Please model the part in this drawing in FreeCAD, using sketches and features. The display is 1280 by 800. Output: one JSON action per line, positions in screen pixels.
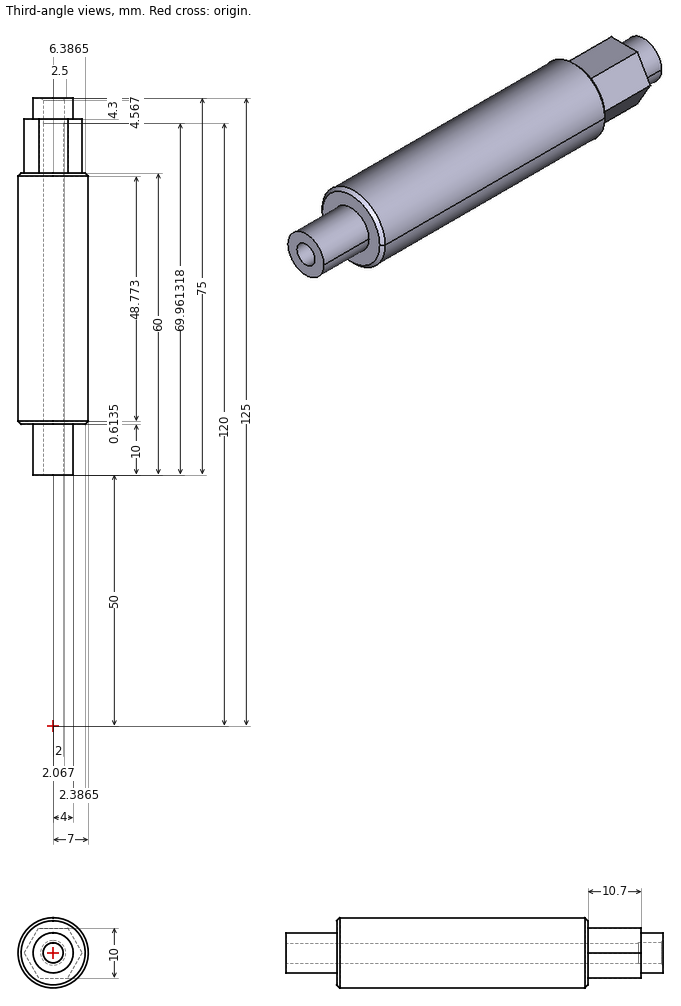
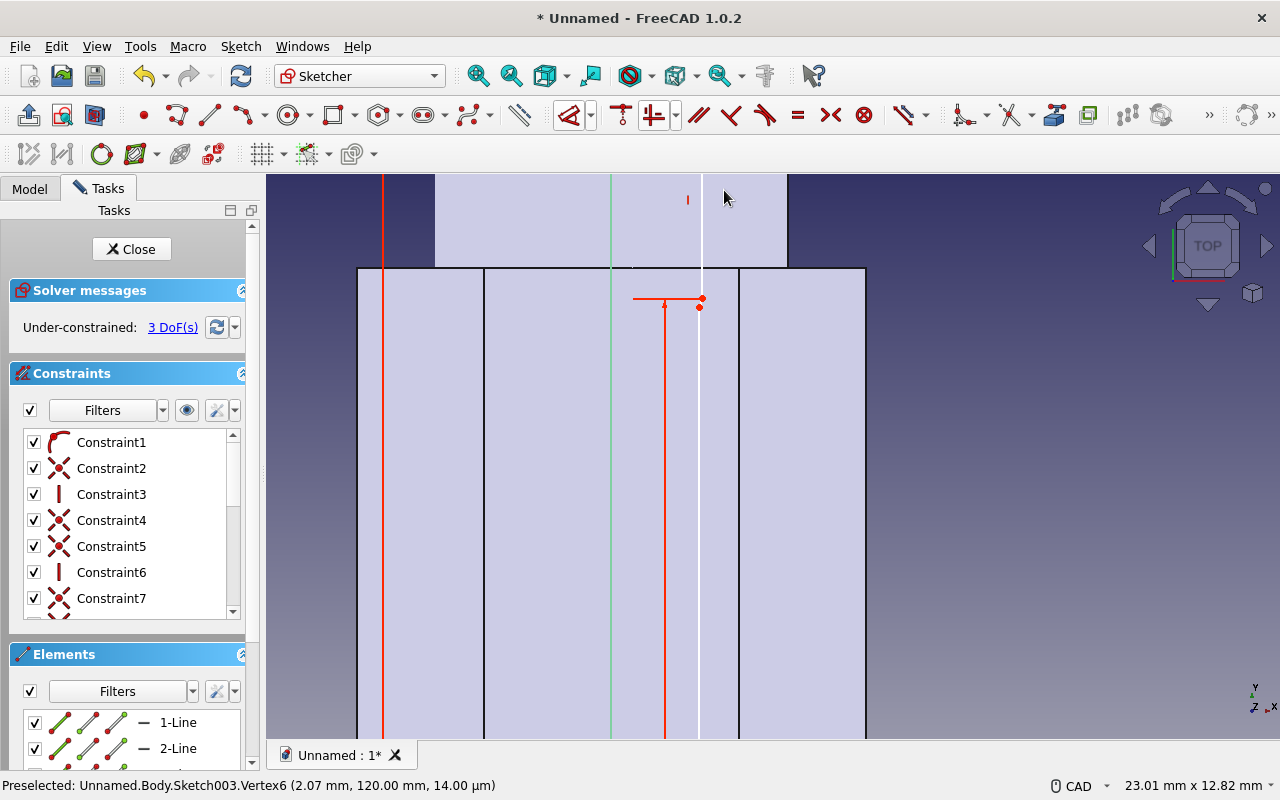
{"action": "scroll", "coordinate": [707, 303], "scroll_direction": "down", "scroll_amount": 14}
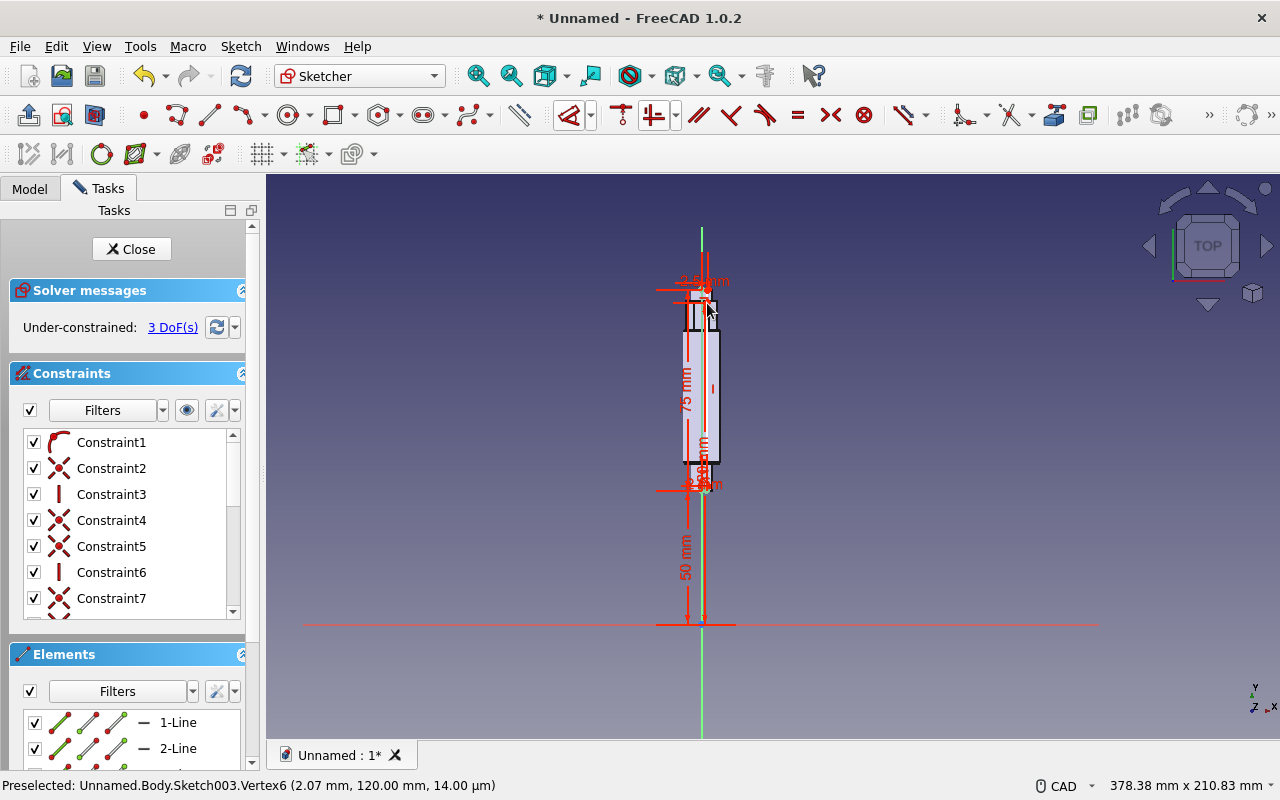
{"action": "scroll", "coordinate": [707, 299], "scroll_direction": "up", "scroll_amount": 7}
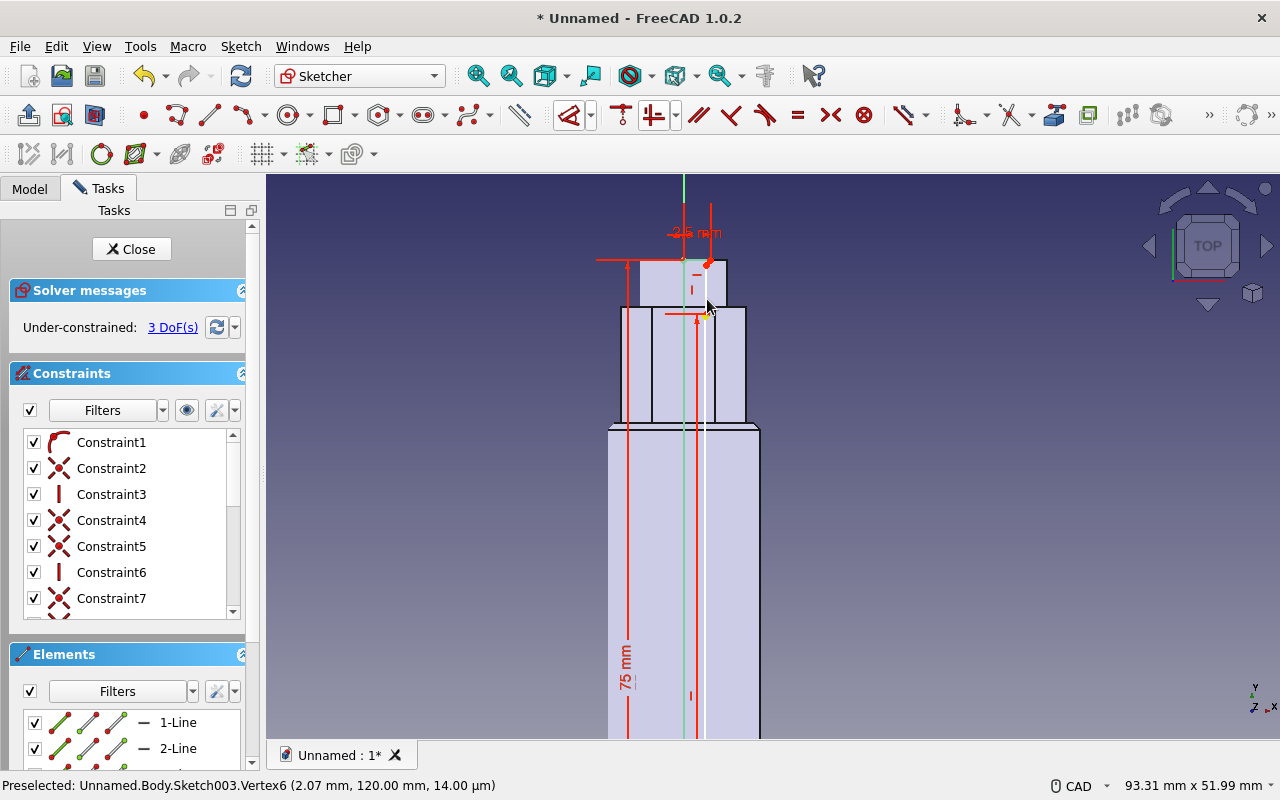
{"action": "left_click", "coordinate": [706, 300]}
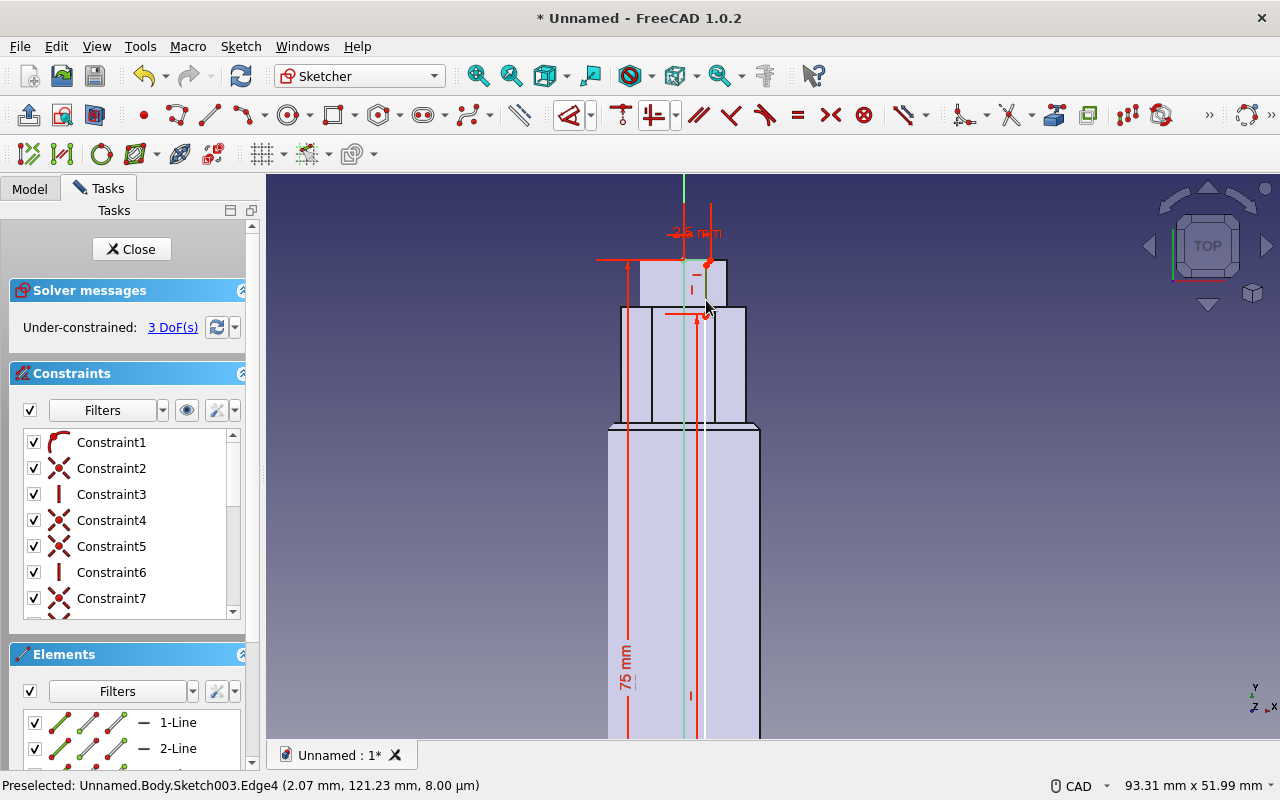
{"action": "left_click", "coordinate": [590, 116]}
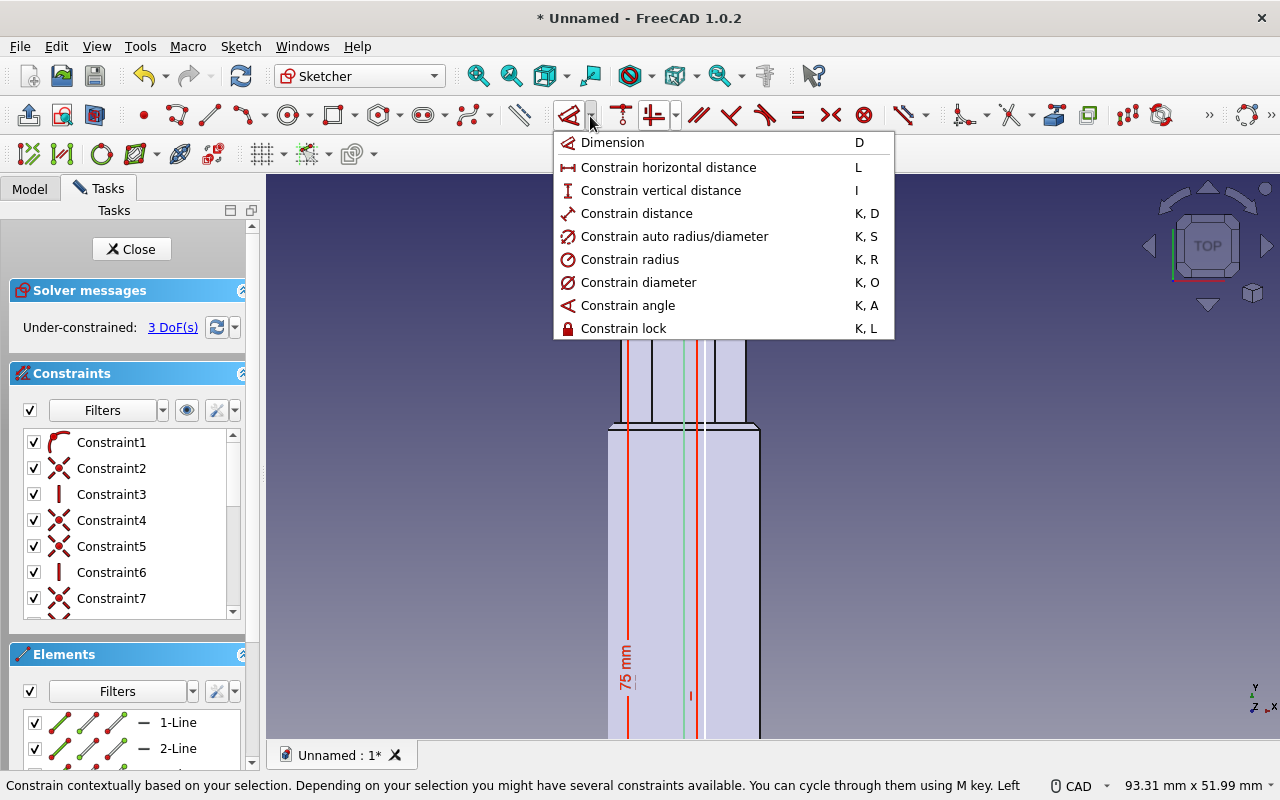
{"action": "left_click", "coordinate": [724, 190]}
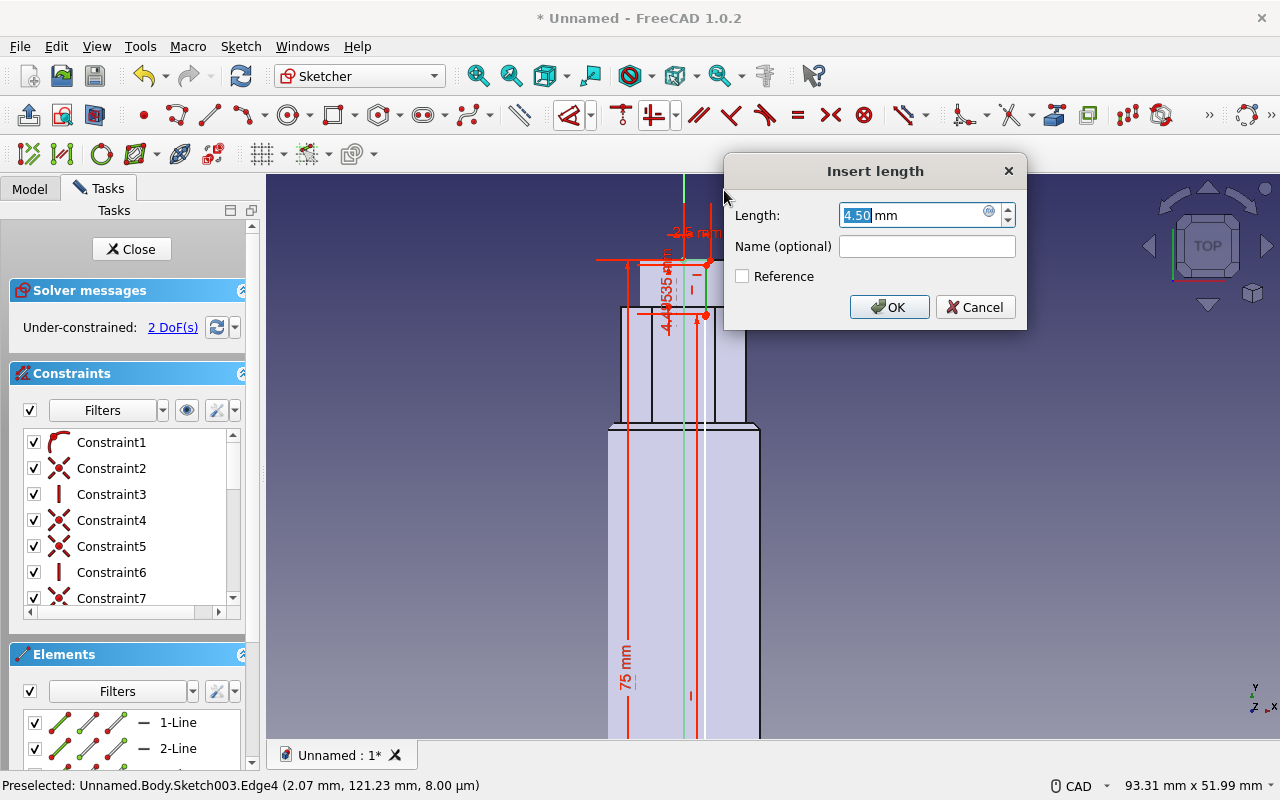
{"action": "type", "text": "4.567"}
{"action": "key", "text": "Return"}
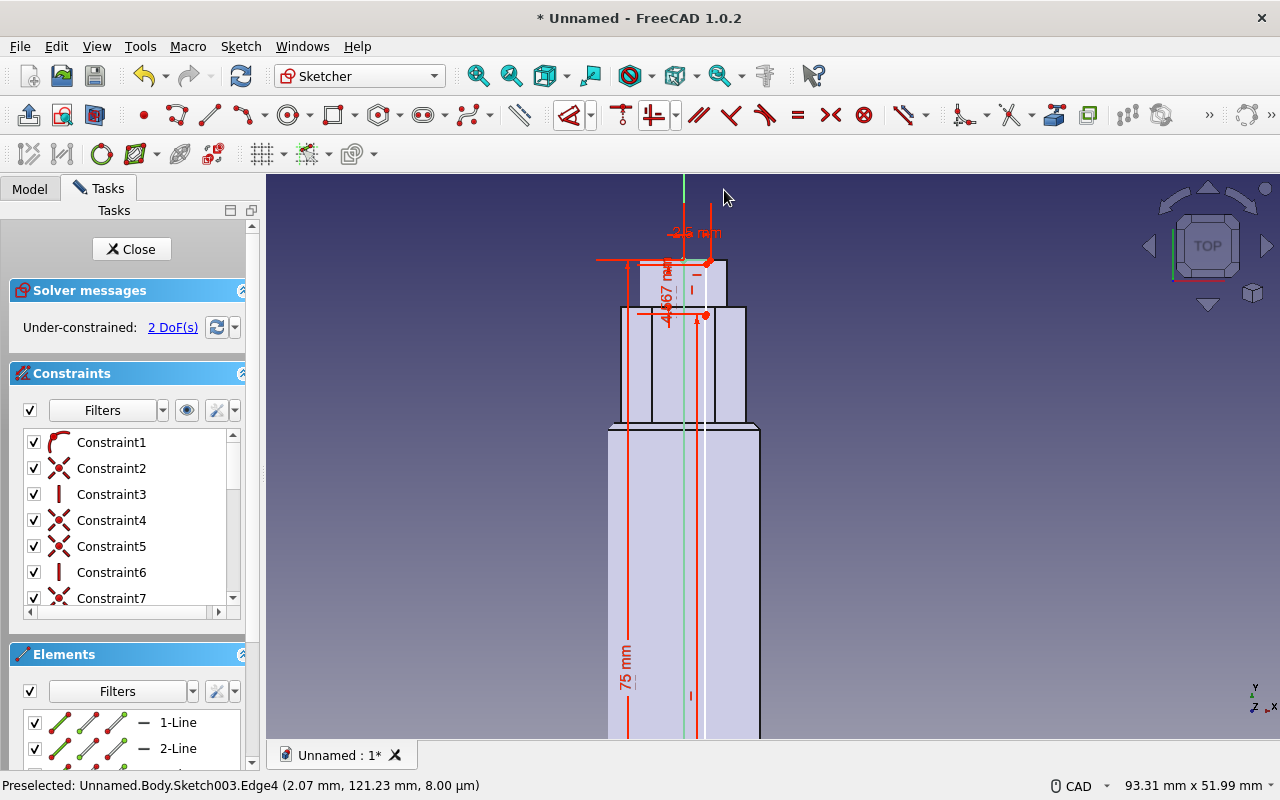
{"action": "scroll", "coordinate": [706, 314], "scroll_direction": "up", "scroll_amount": 7}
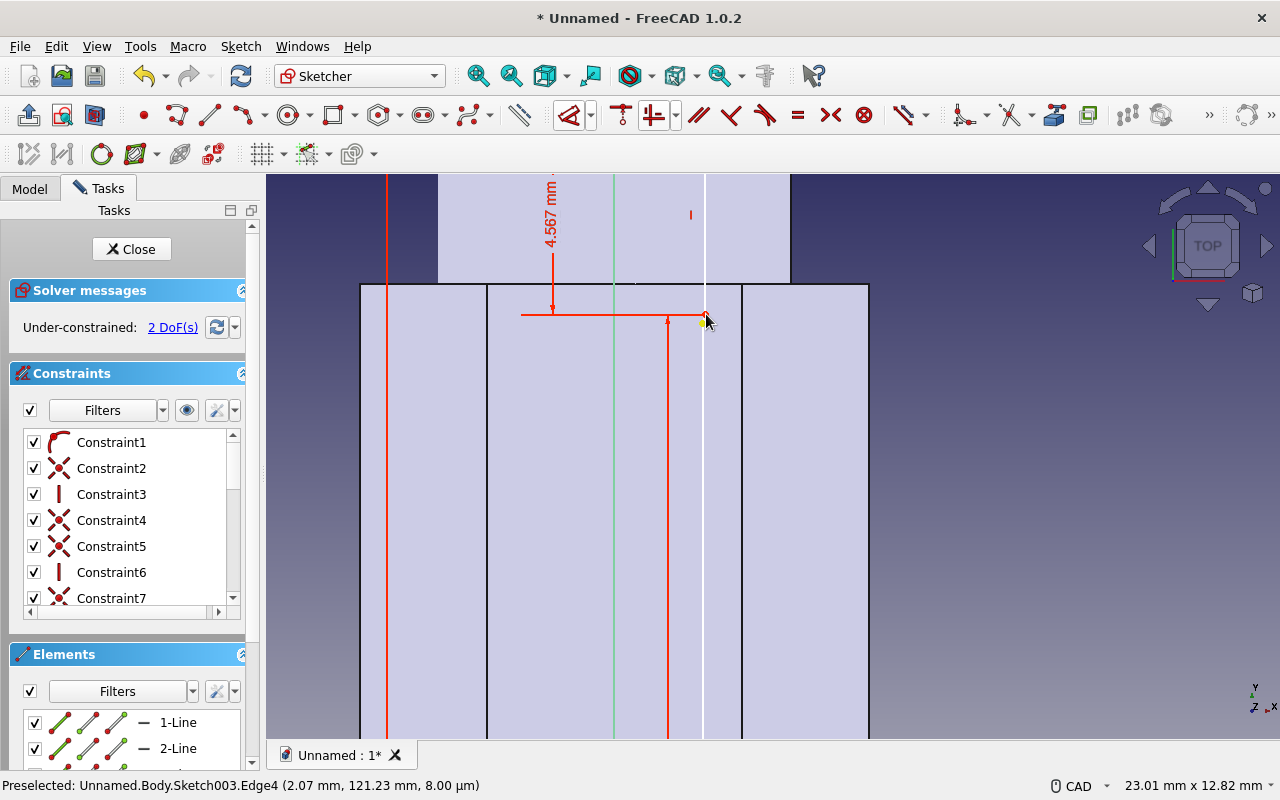
{"action": "left_click", "coordinate": [705, 315]}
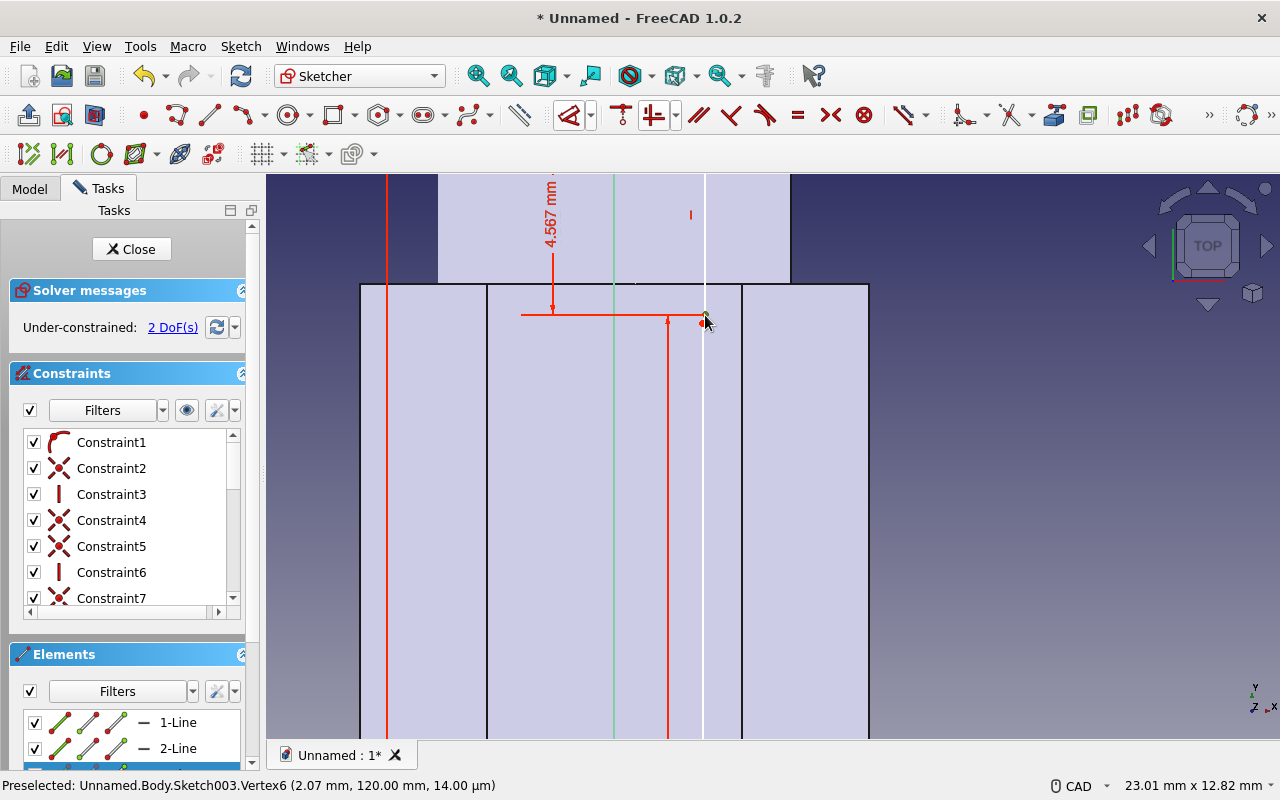
{"action": "left_click", "coordinate": [590, 116]}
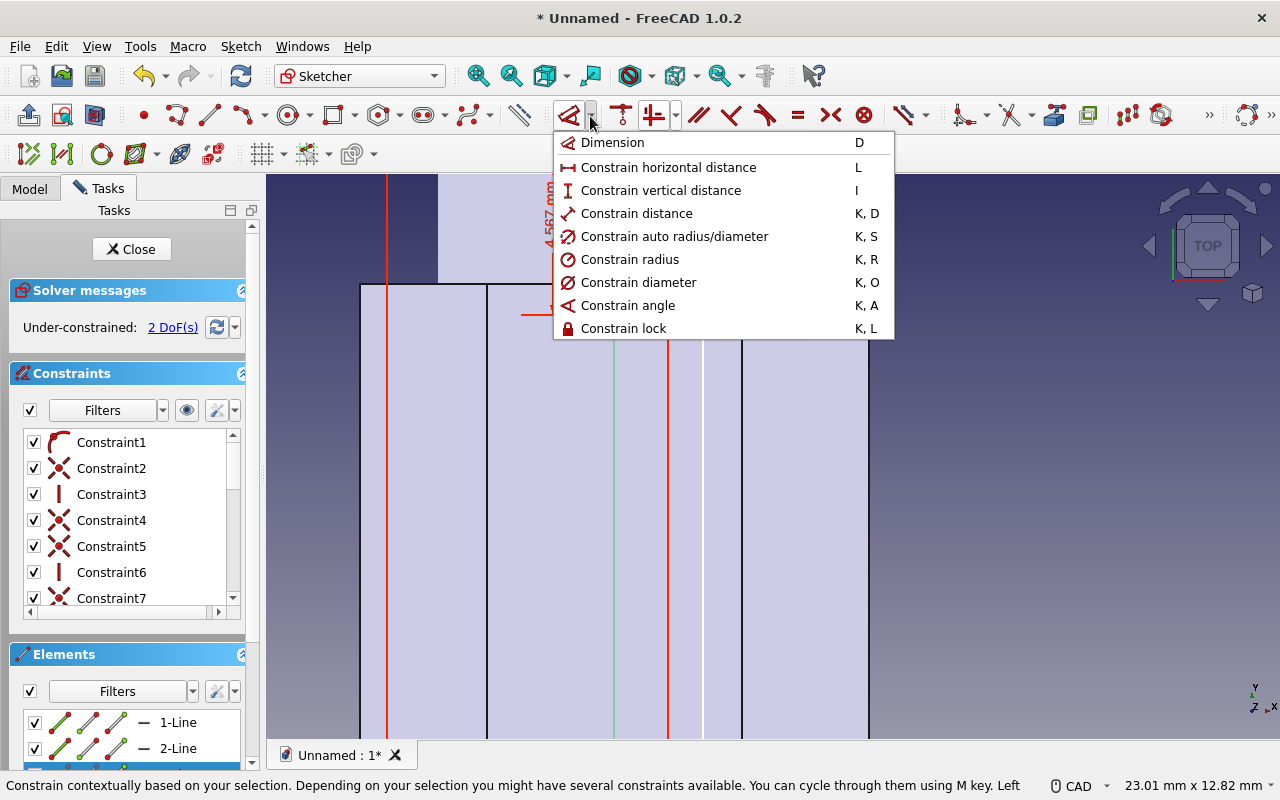
{"action": "left_click", "coordinate": [724, 168]}